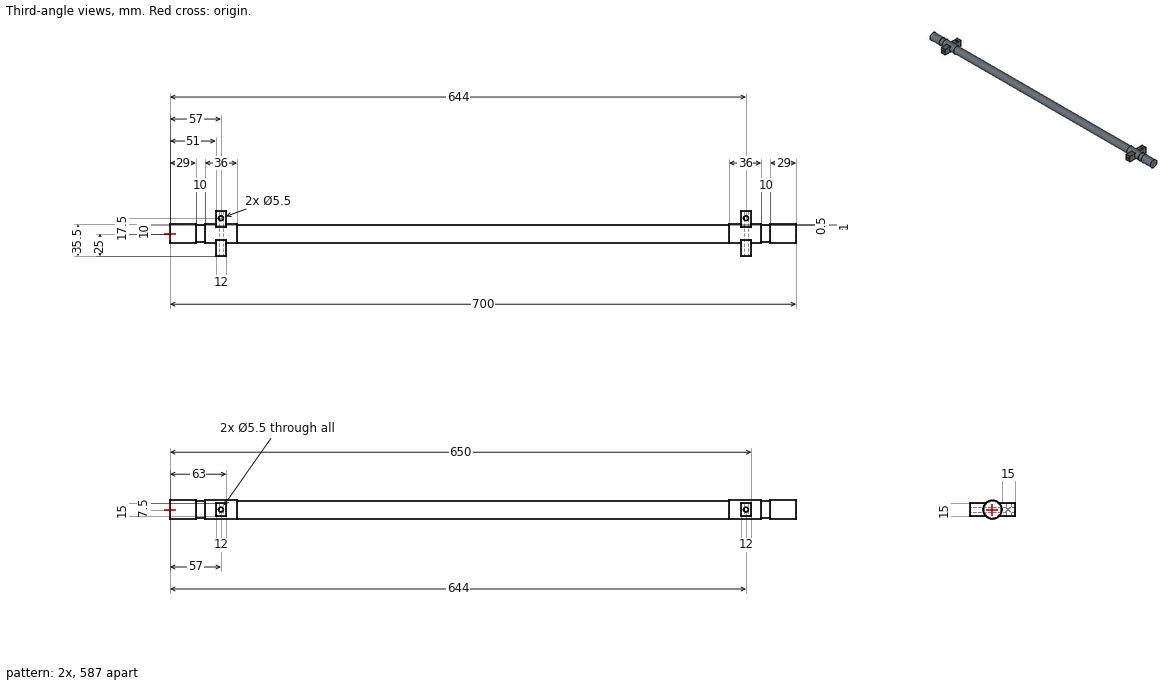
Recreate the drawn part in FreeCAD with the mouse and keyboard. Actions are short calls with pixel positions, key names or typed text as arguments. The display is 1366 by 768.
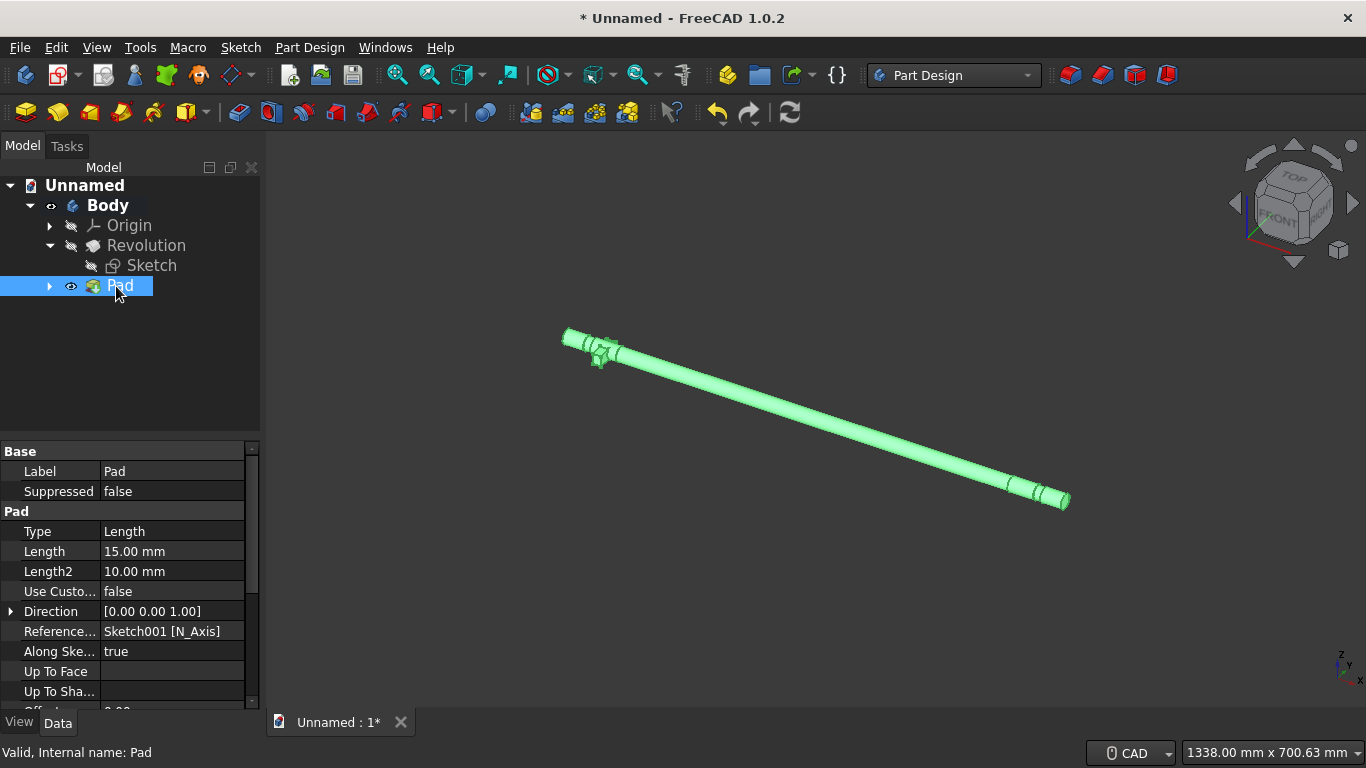
click(564, 112)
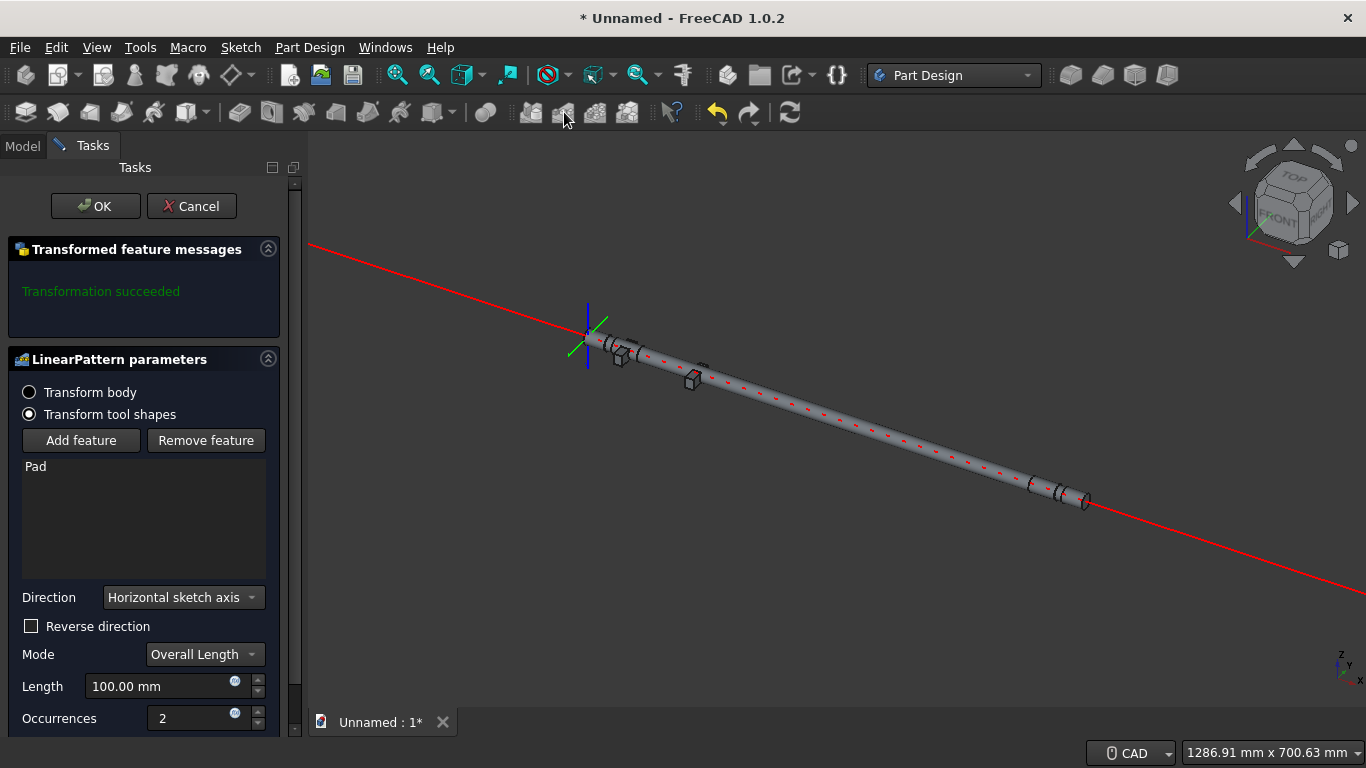
click(184, 598)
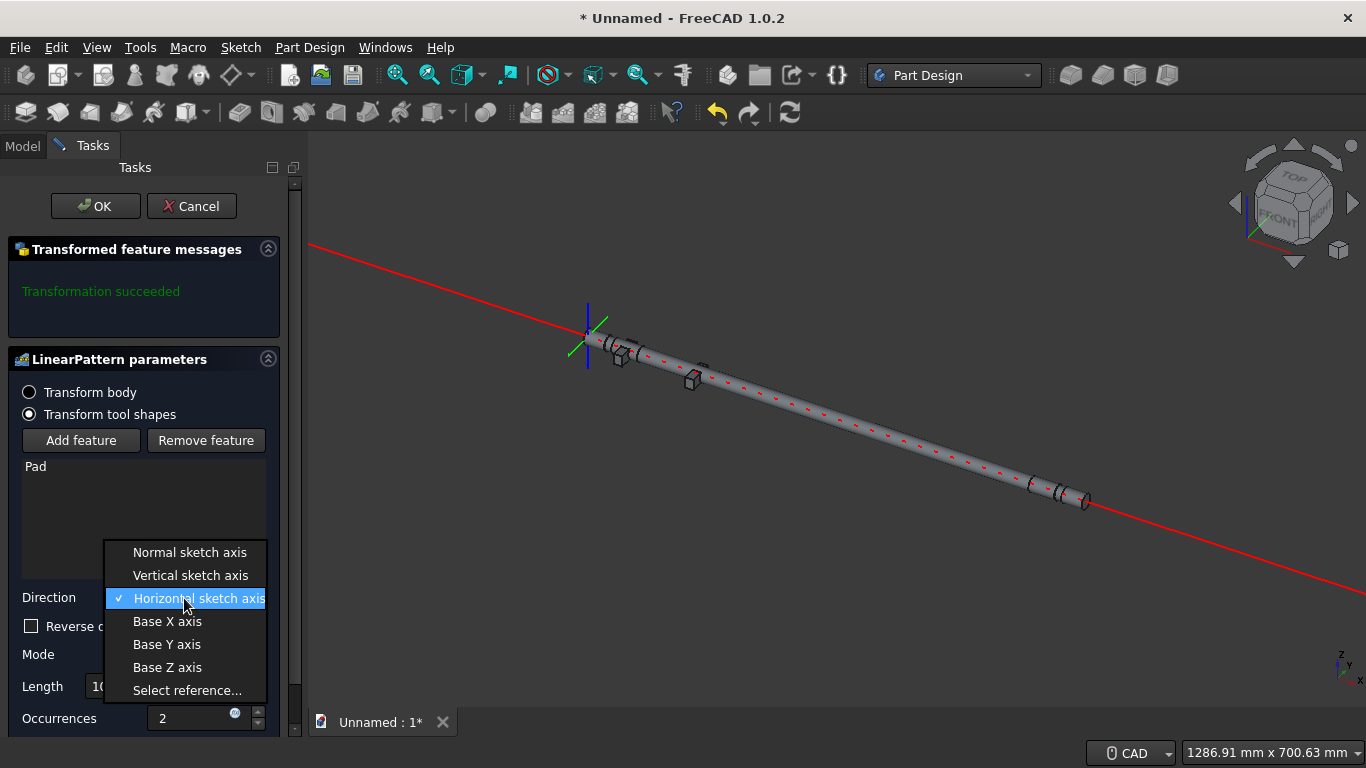
click(184, 622)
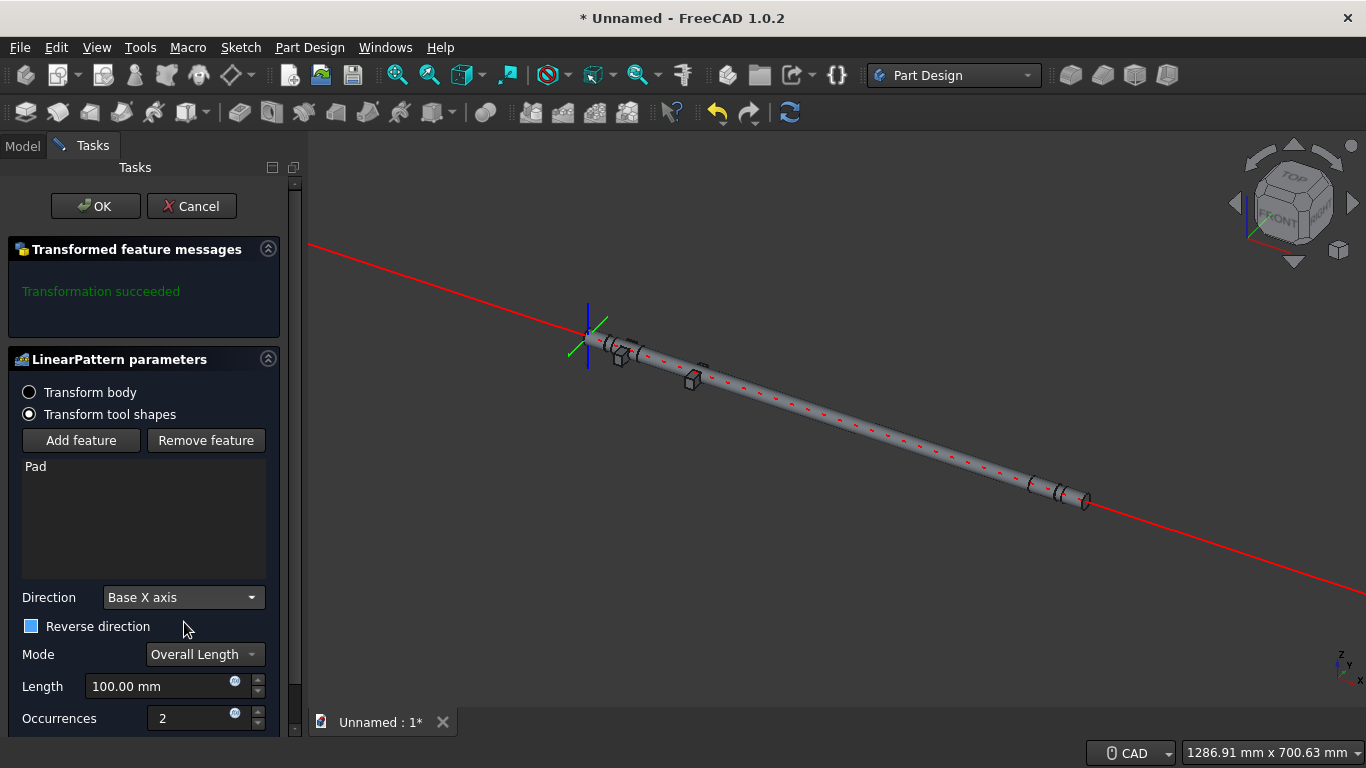
click(206, 654)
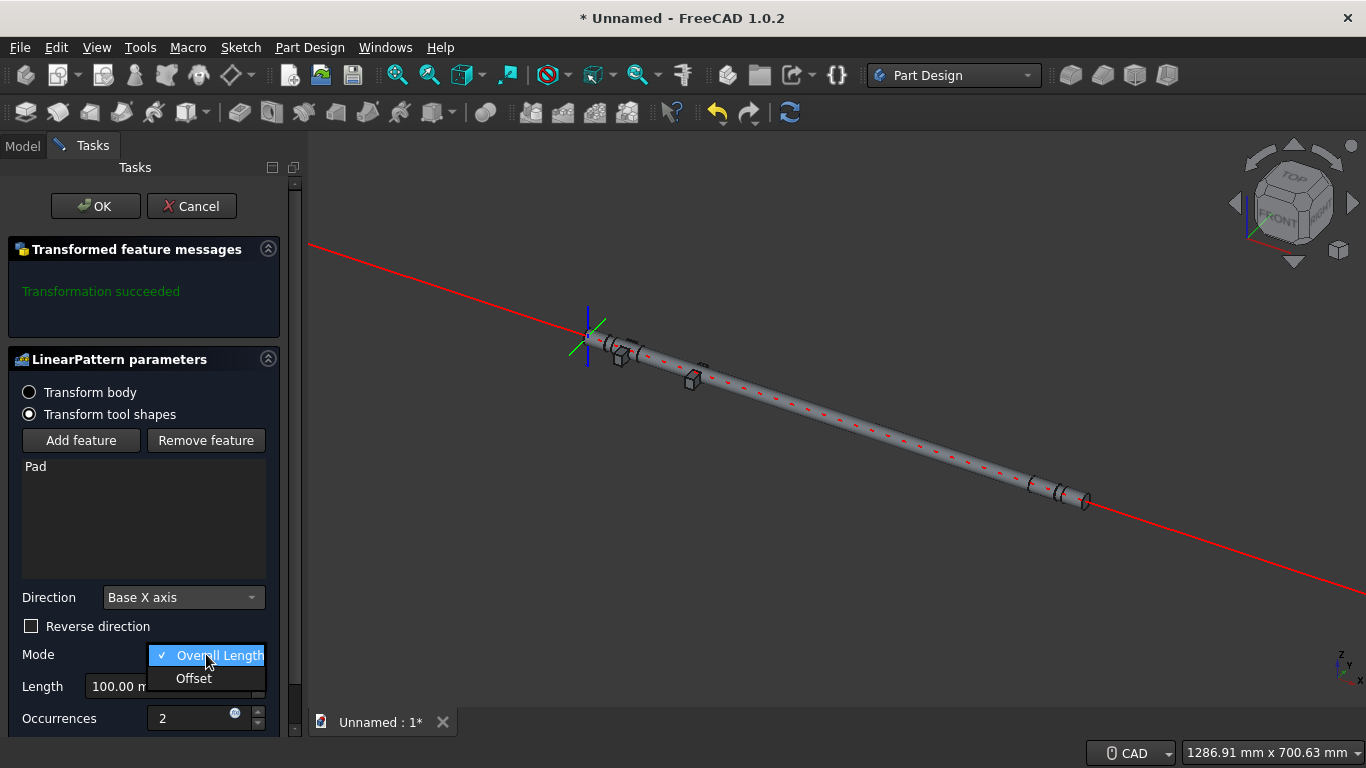
click(206, 678)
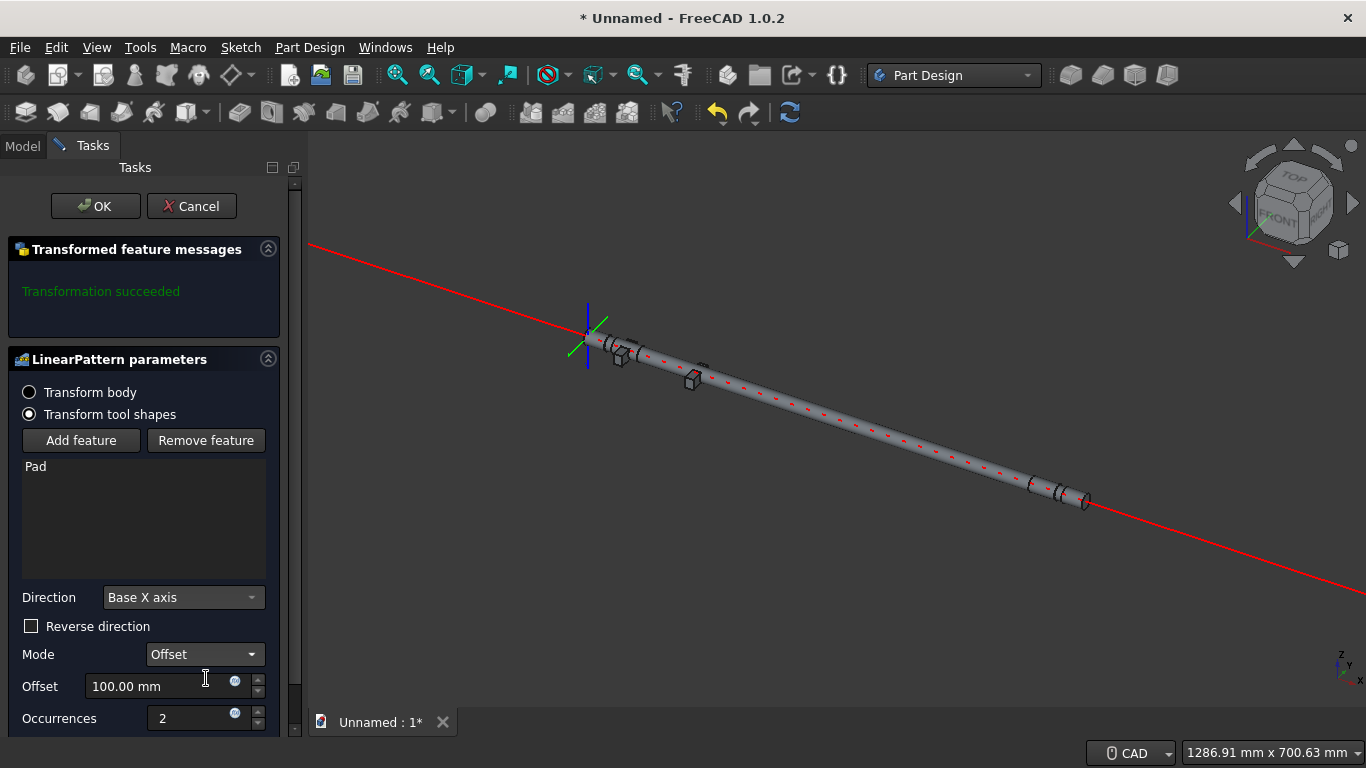
triple_click(168, 686)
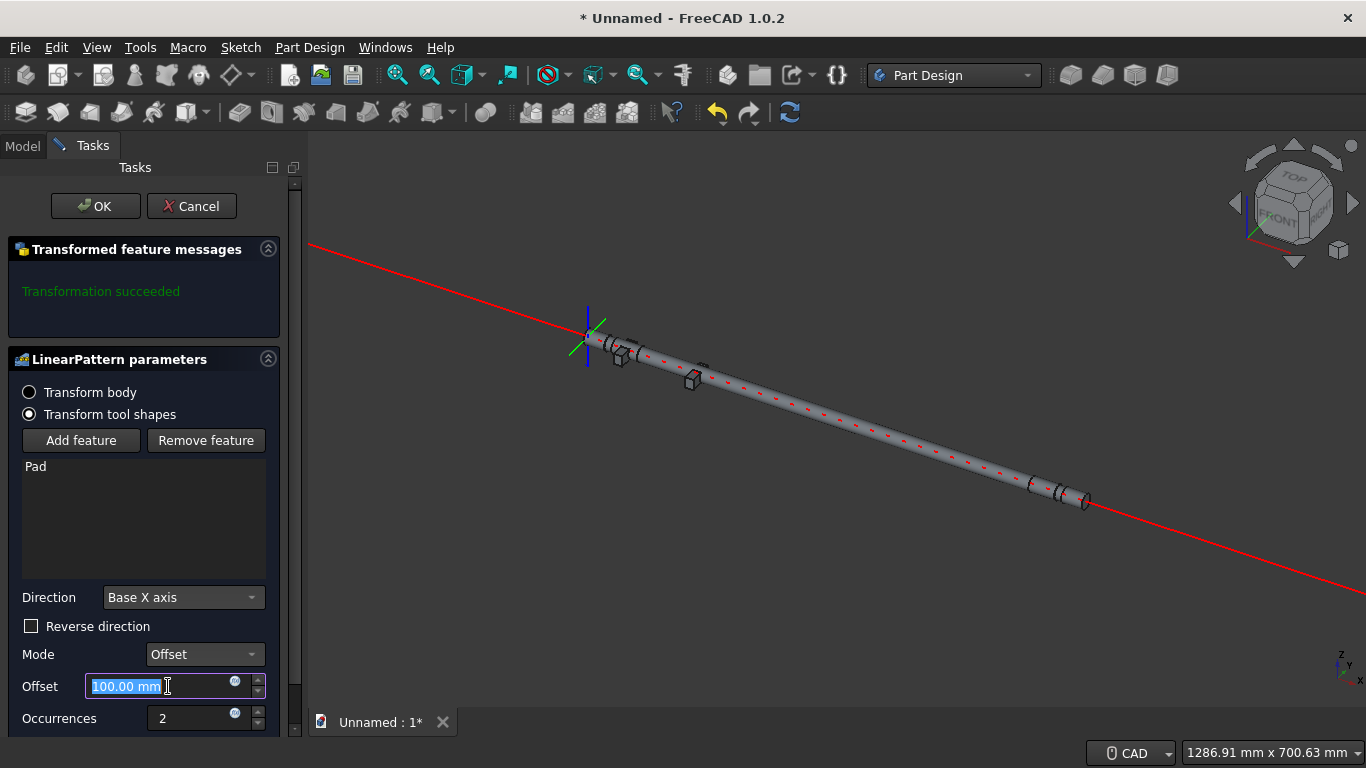
text(587)
key(Tab)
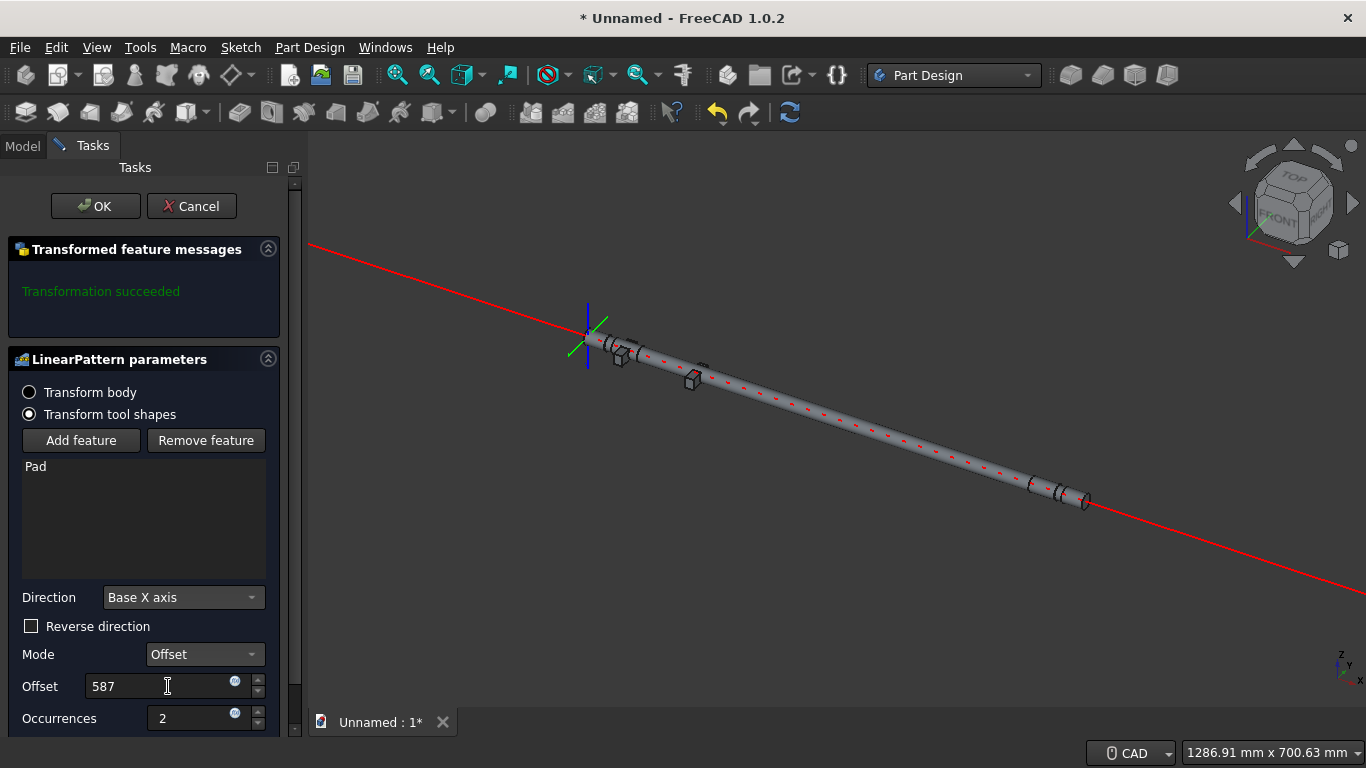
triple_click(198, 718)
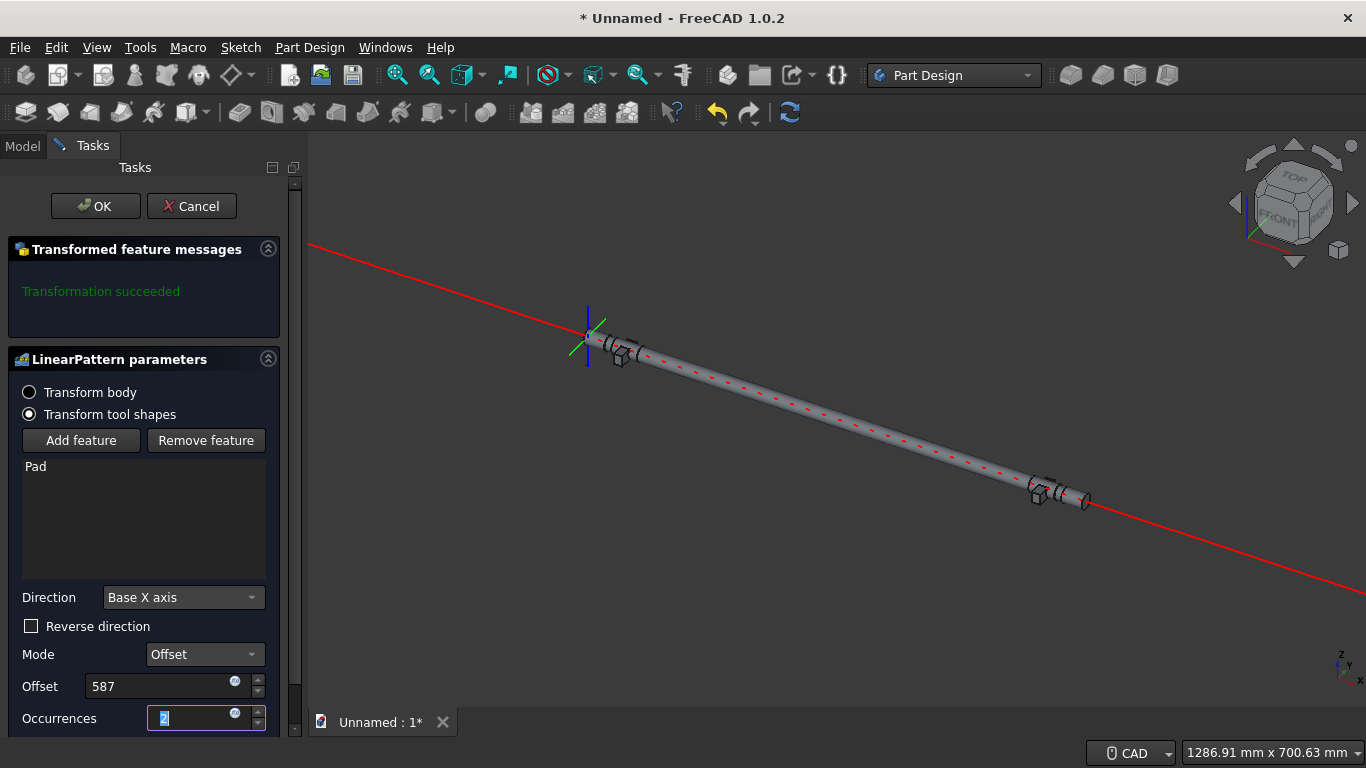
text(2)
key(Tab)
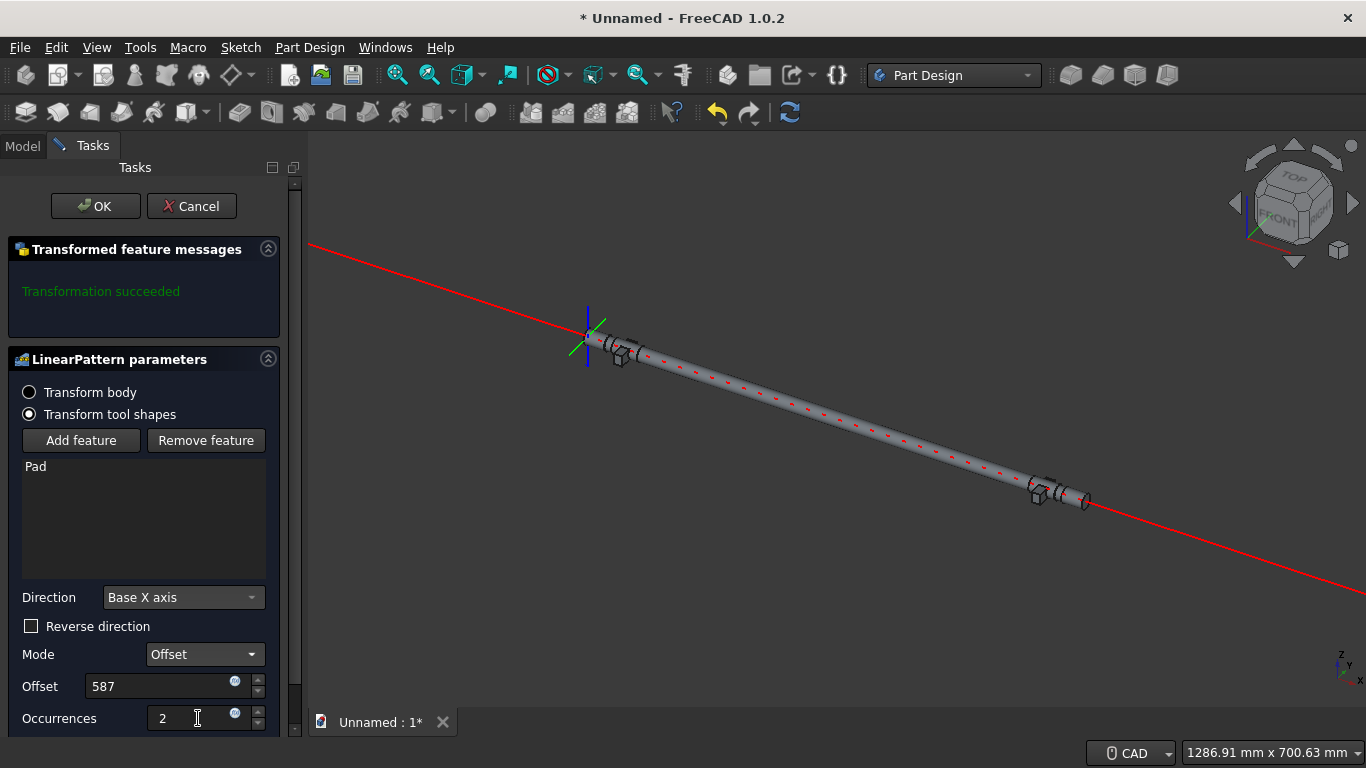
click(96, 206)